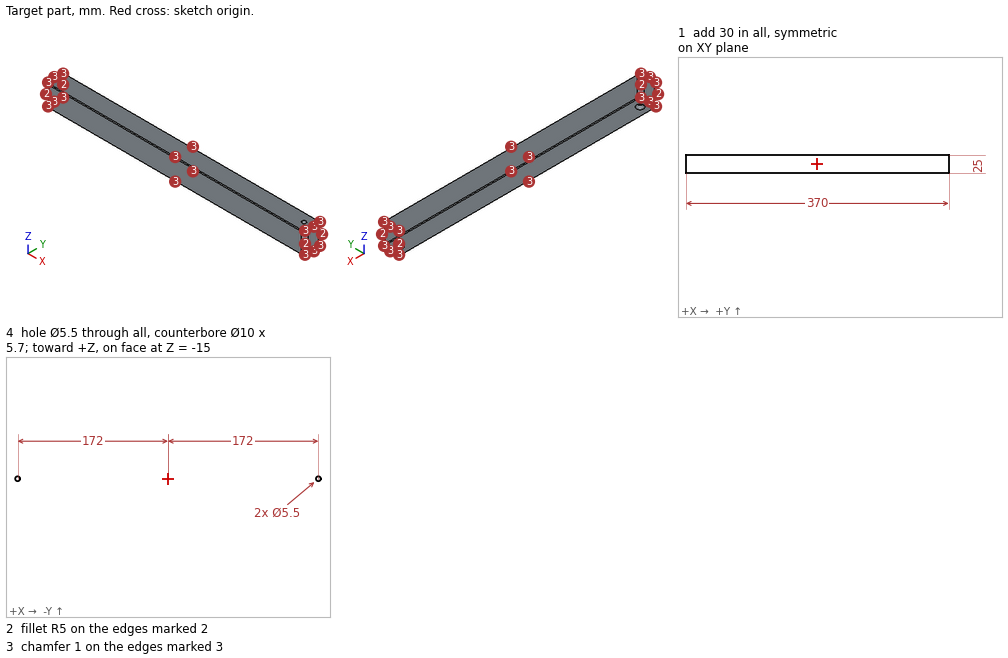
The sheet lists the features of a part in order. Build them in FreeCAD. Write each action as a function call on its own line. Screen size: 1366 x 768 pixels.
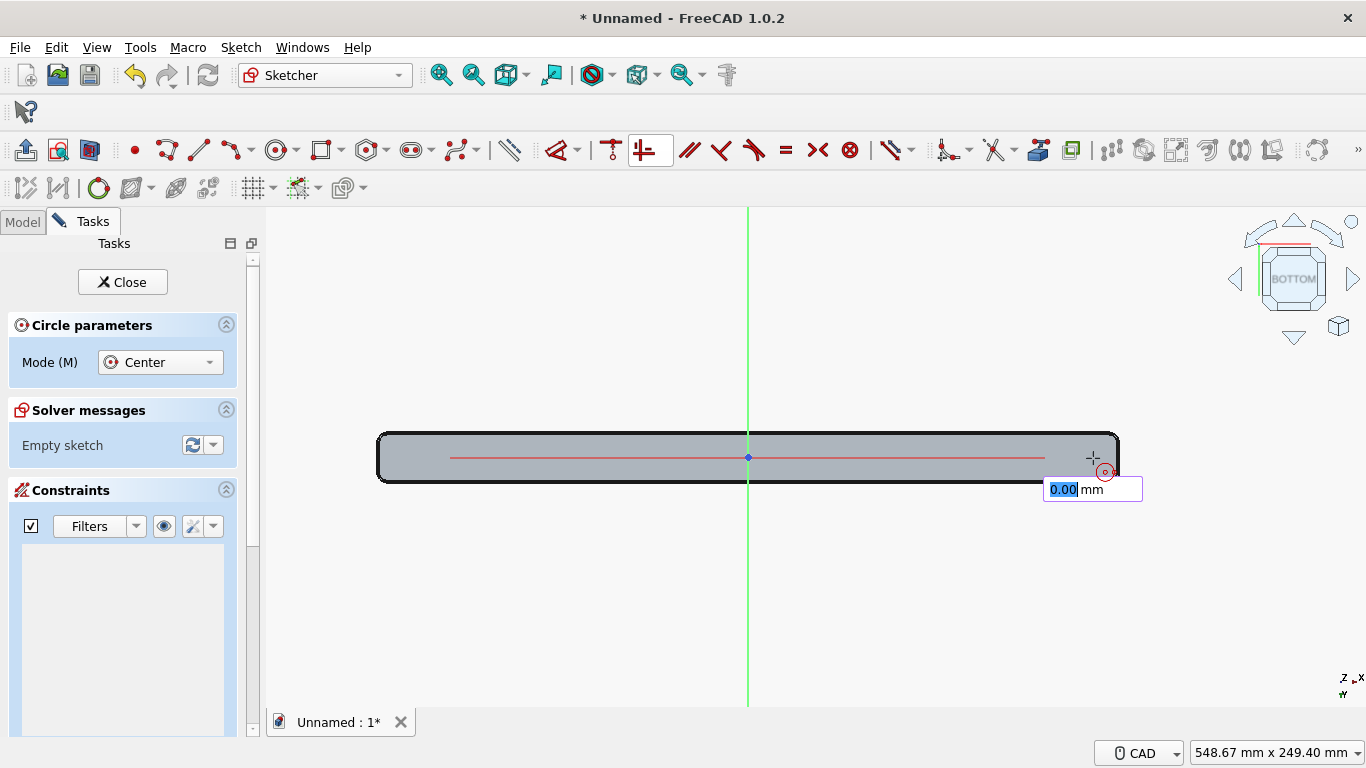
scroll(1095, 452, up, 6)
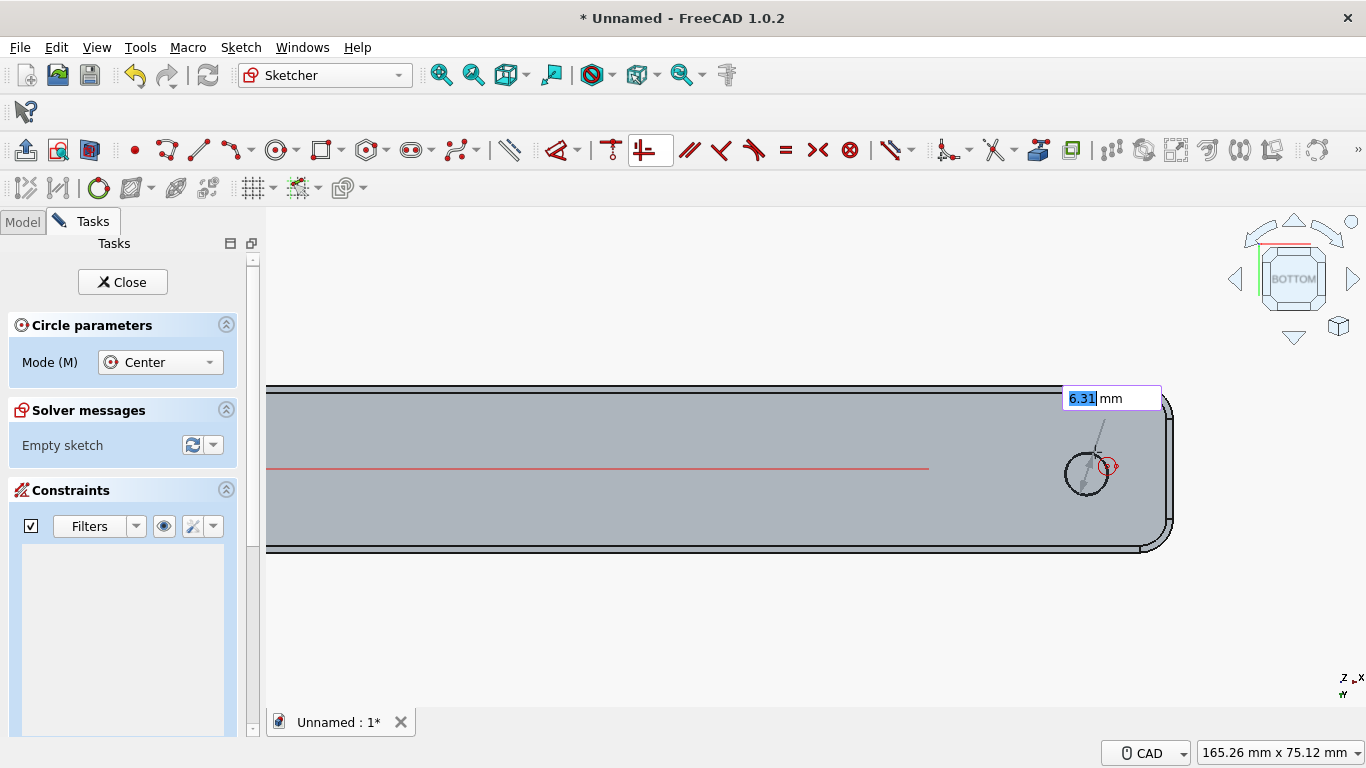
click(1093, 452)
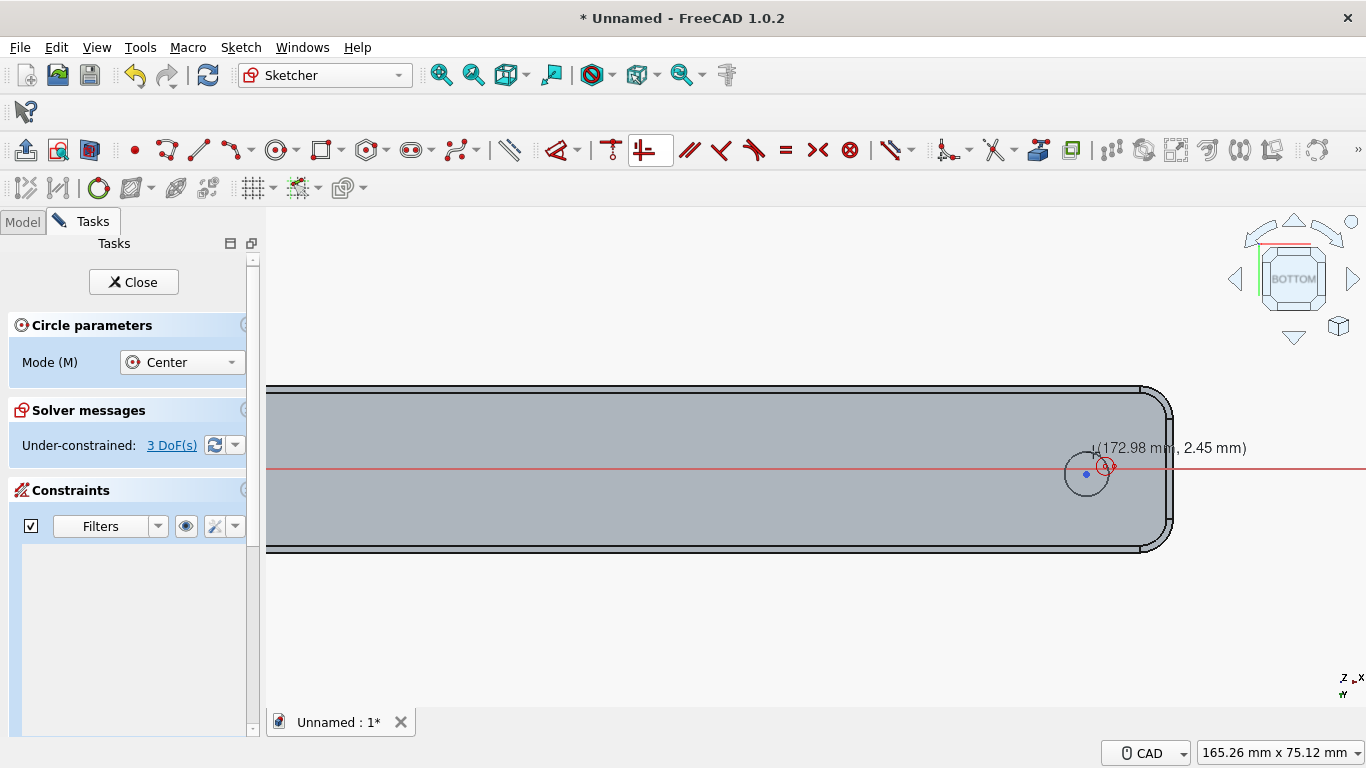
scroll(1095, 452, down, 6)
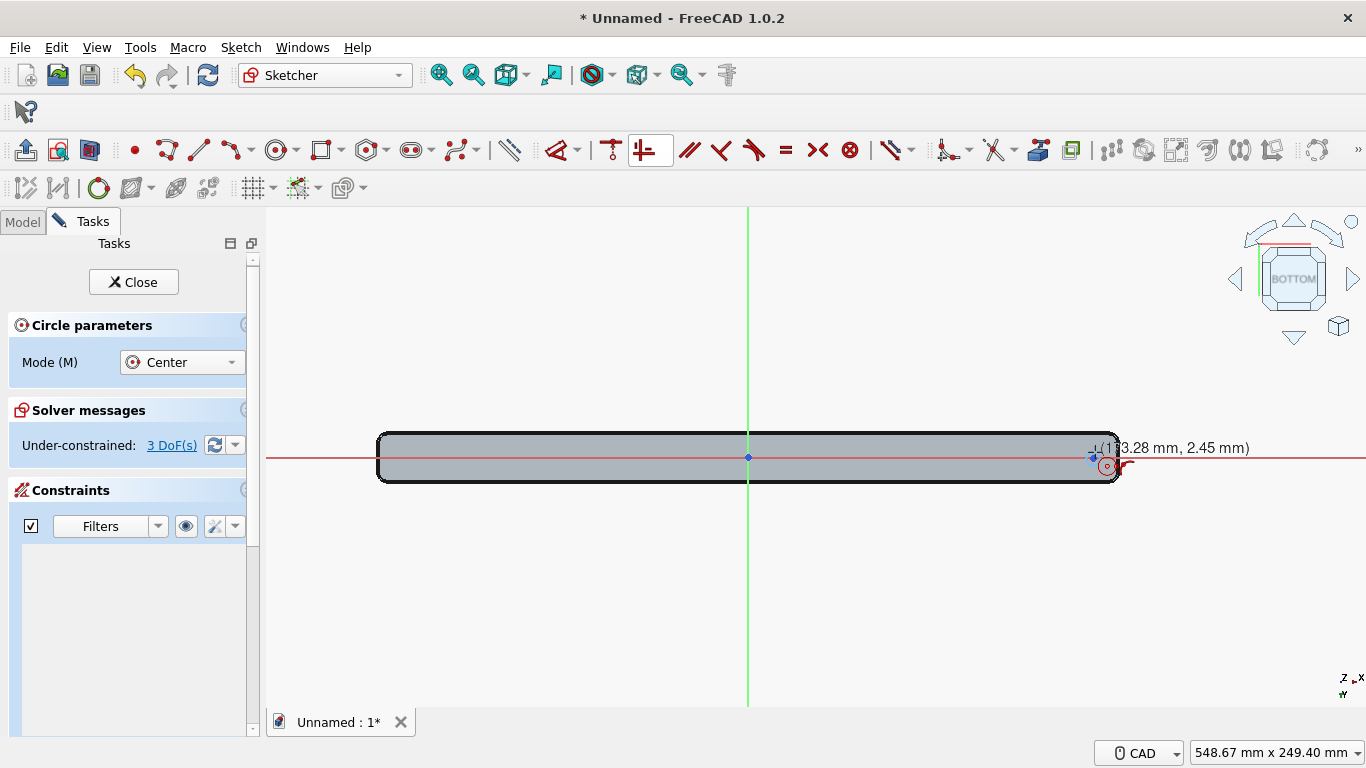
scroll(403, 458, up, 8)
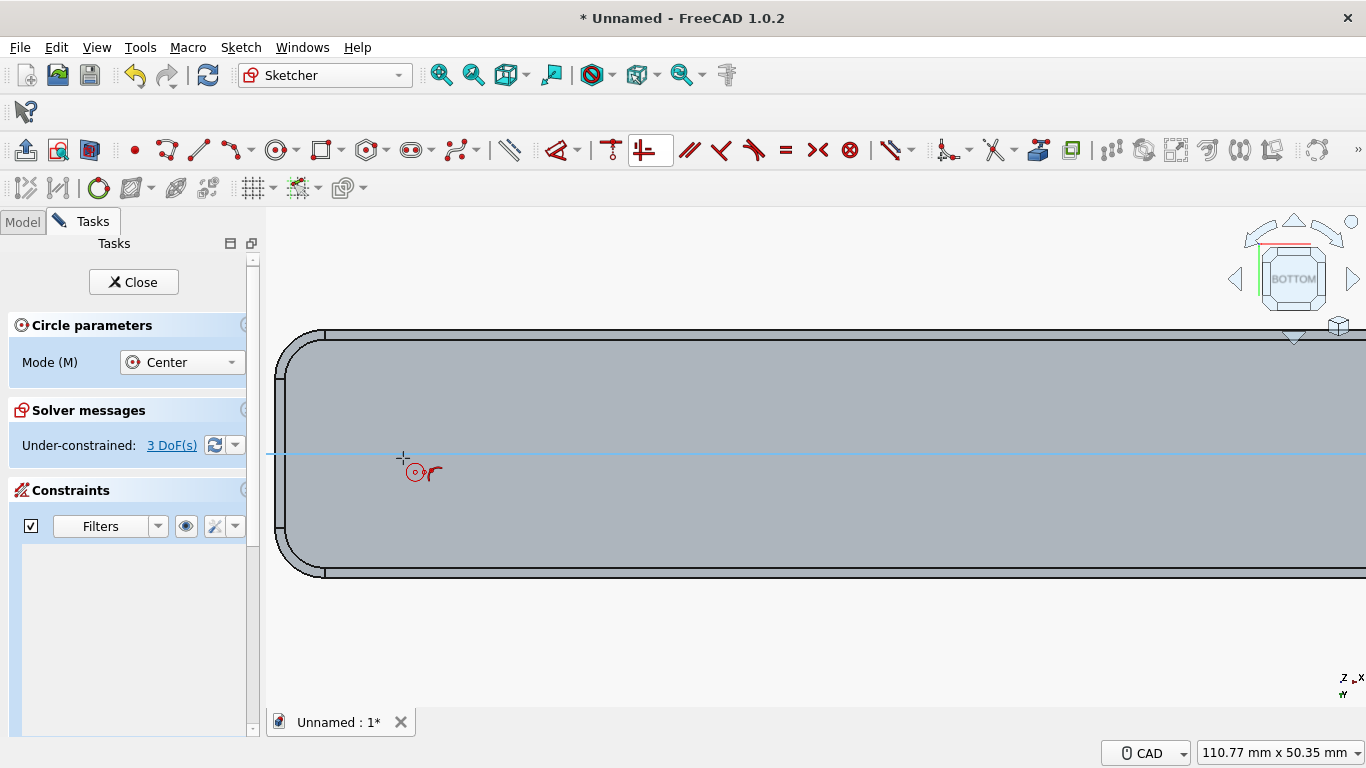
scroll(402, 458, down, 8)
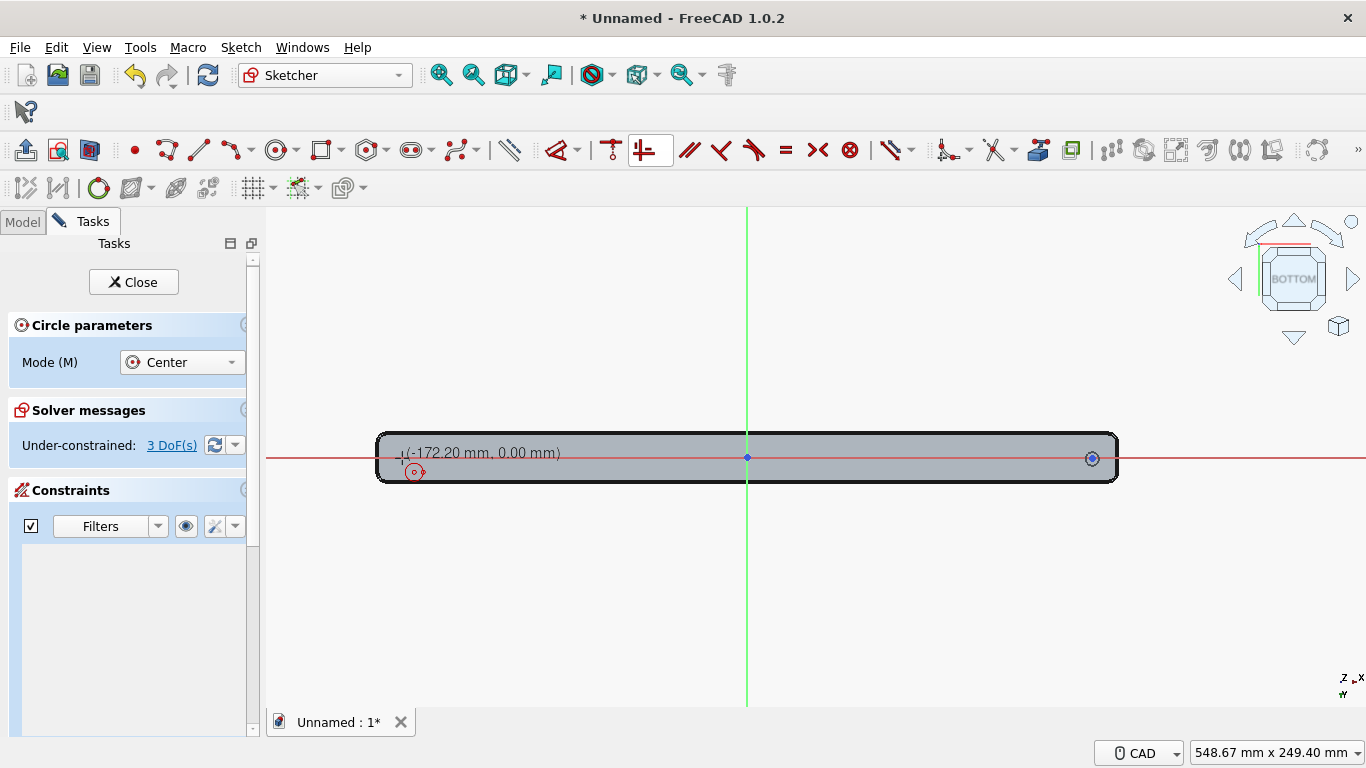
click(402, 458)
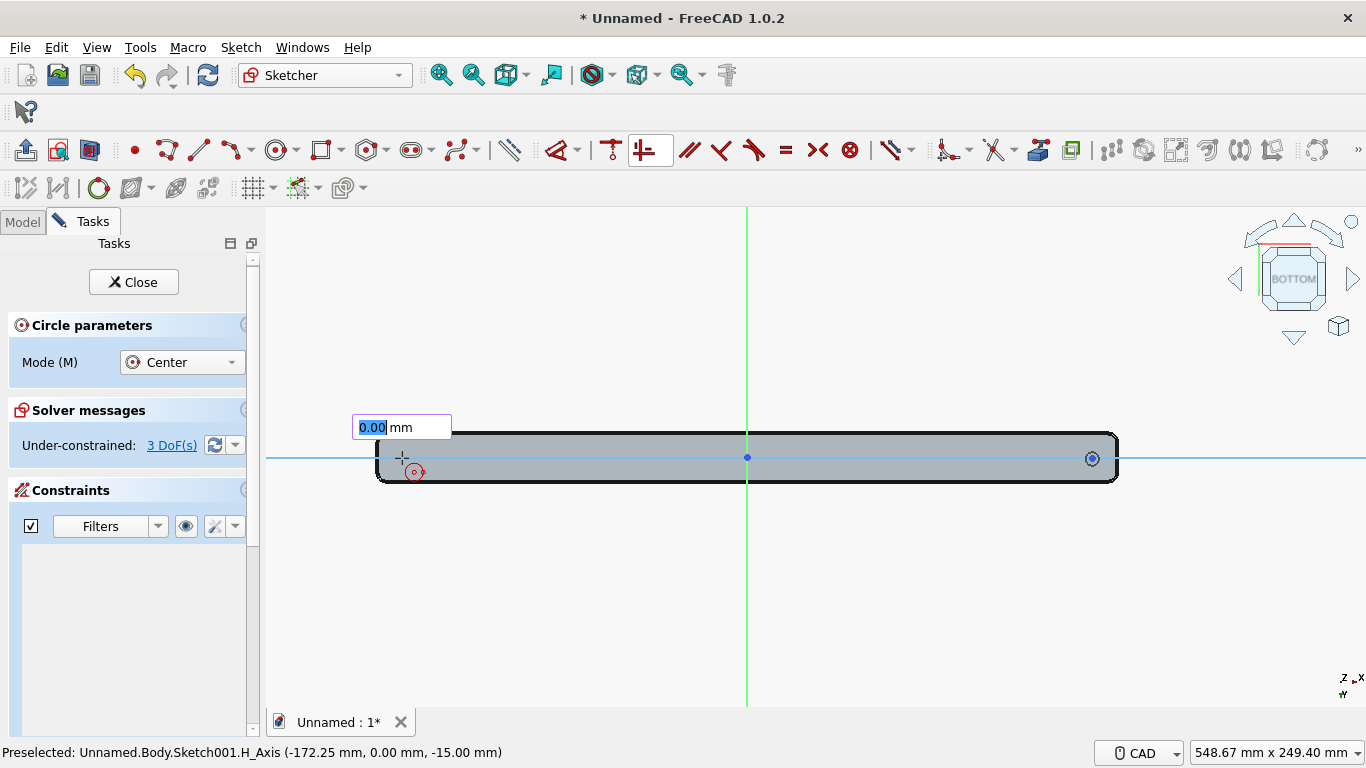
scroll(404, 452, up, 6)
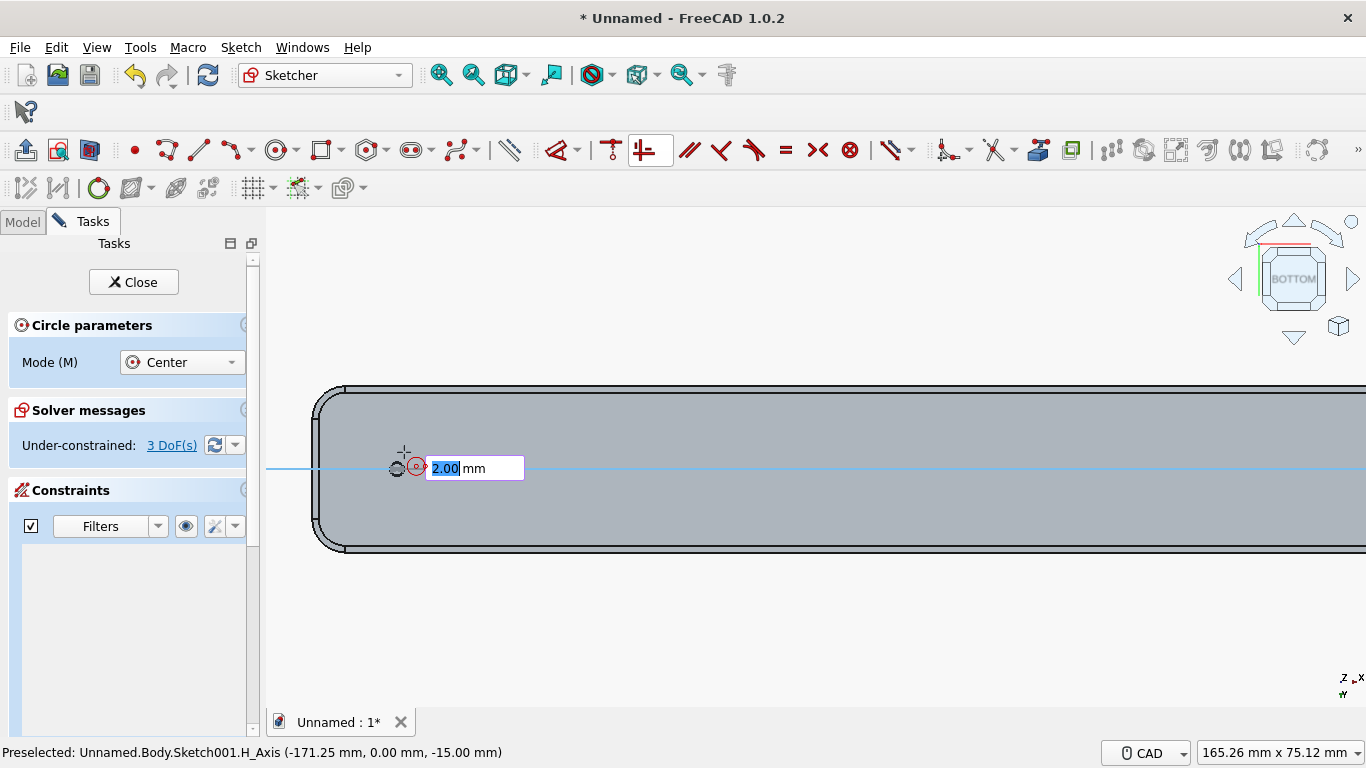
click(405, 452)
key(Escape)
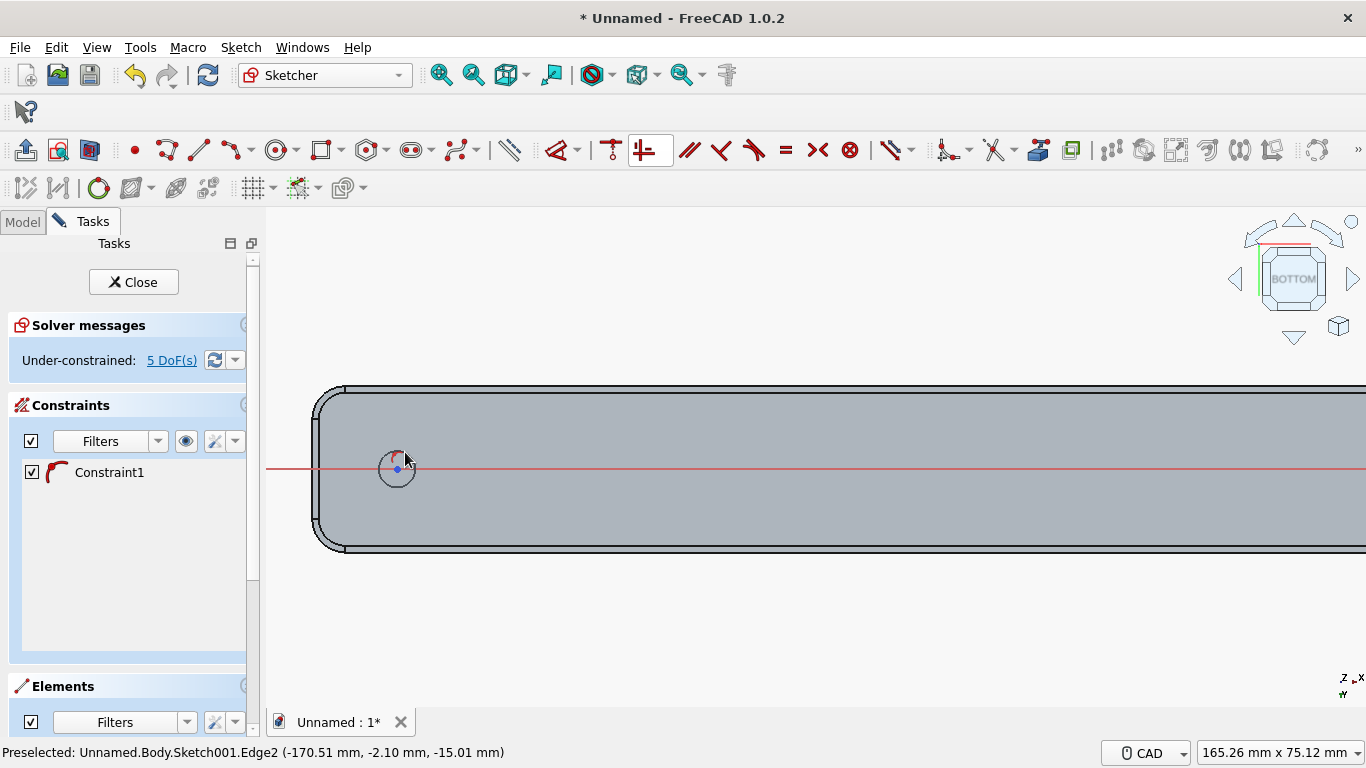
scroll(404, 452, down, 6)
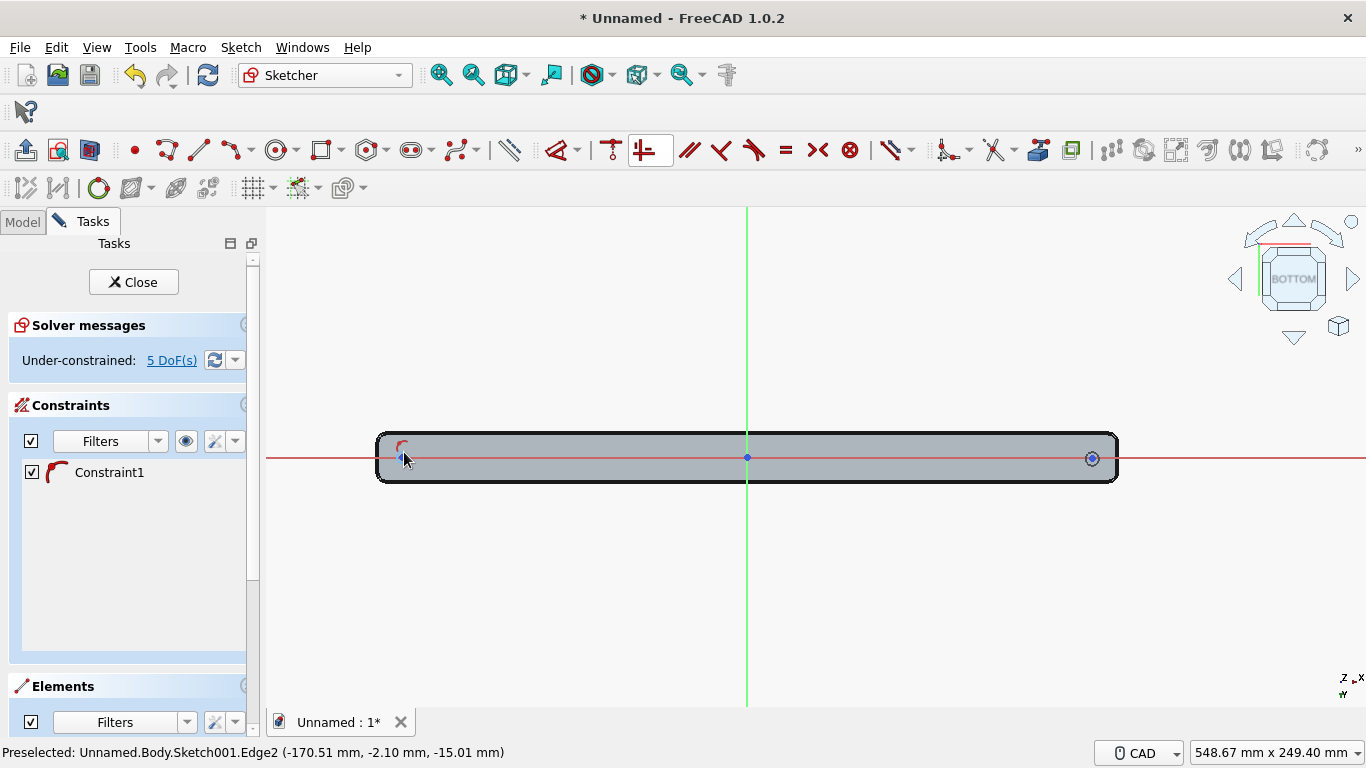
scroll(1097, 454, up, 8)